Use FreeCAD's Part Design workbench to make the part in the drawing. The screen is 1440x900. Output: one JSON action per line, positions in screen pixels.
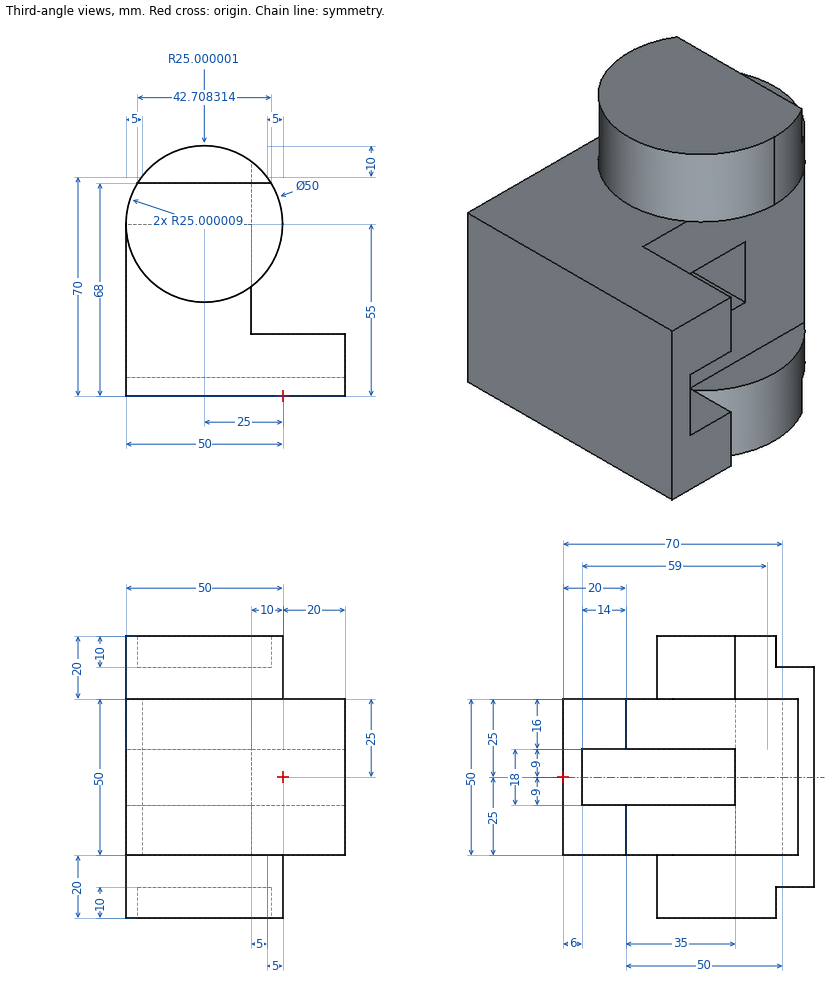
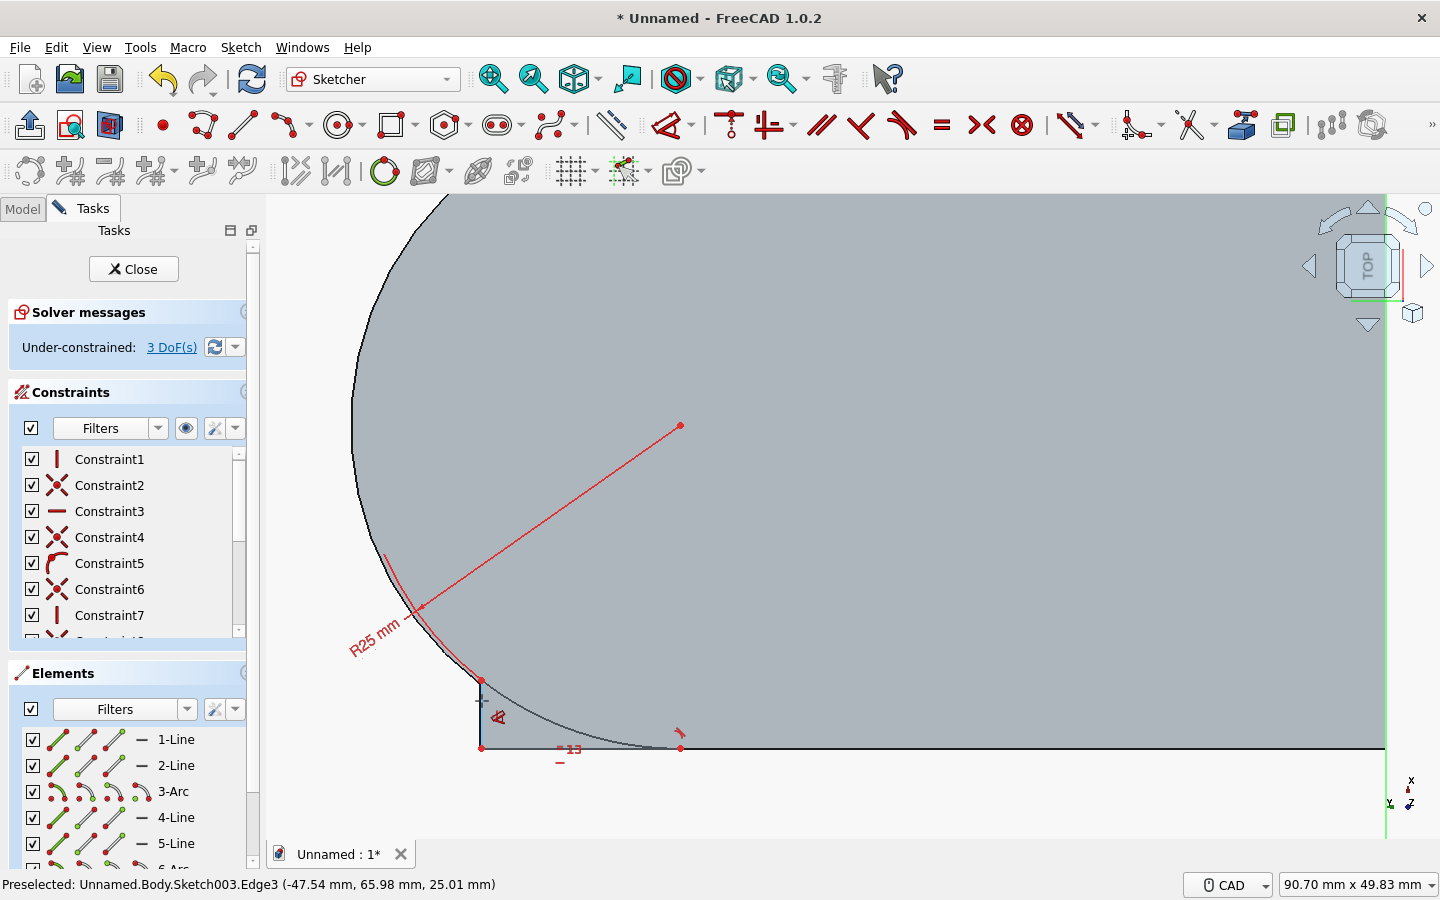
{"action": "left_click", "coordinate": [482, 701]}
{"action": "left_click", "coordinate": [448, 715]}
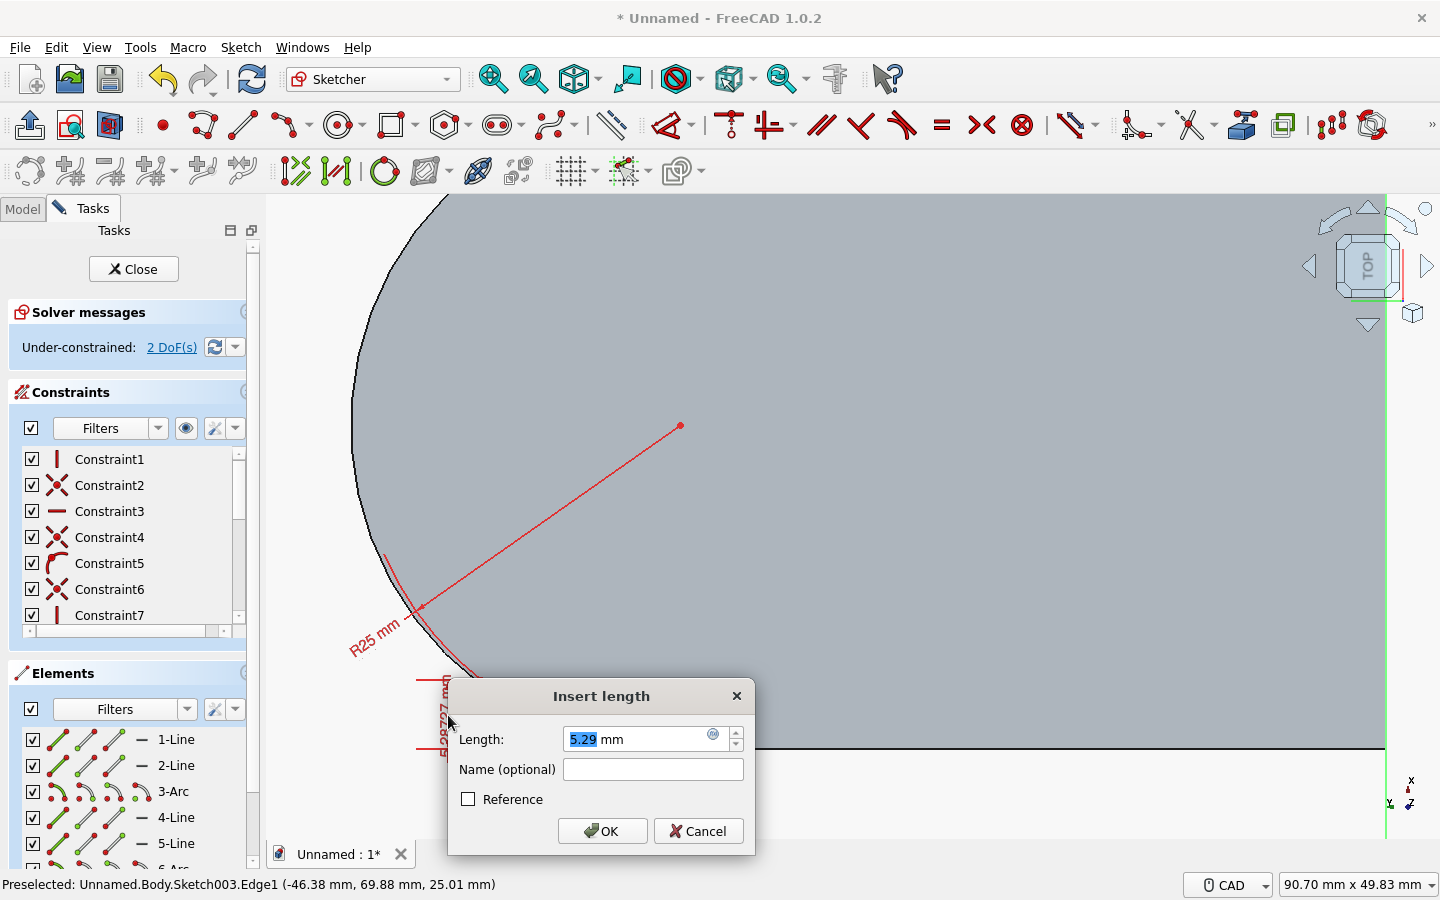
{"action": "type", "text": "5"}
{"action": "key", "text": "Return"}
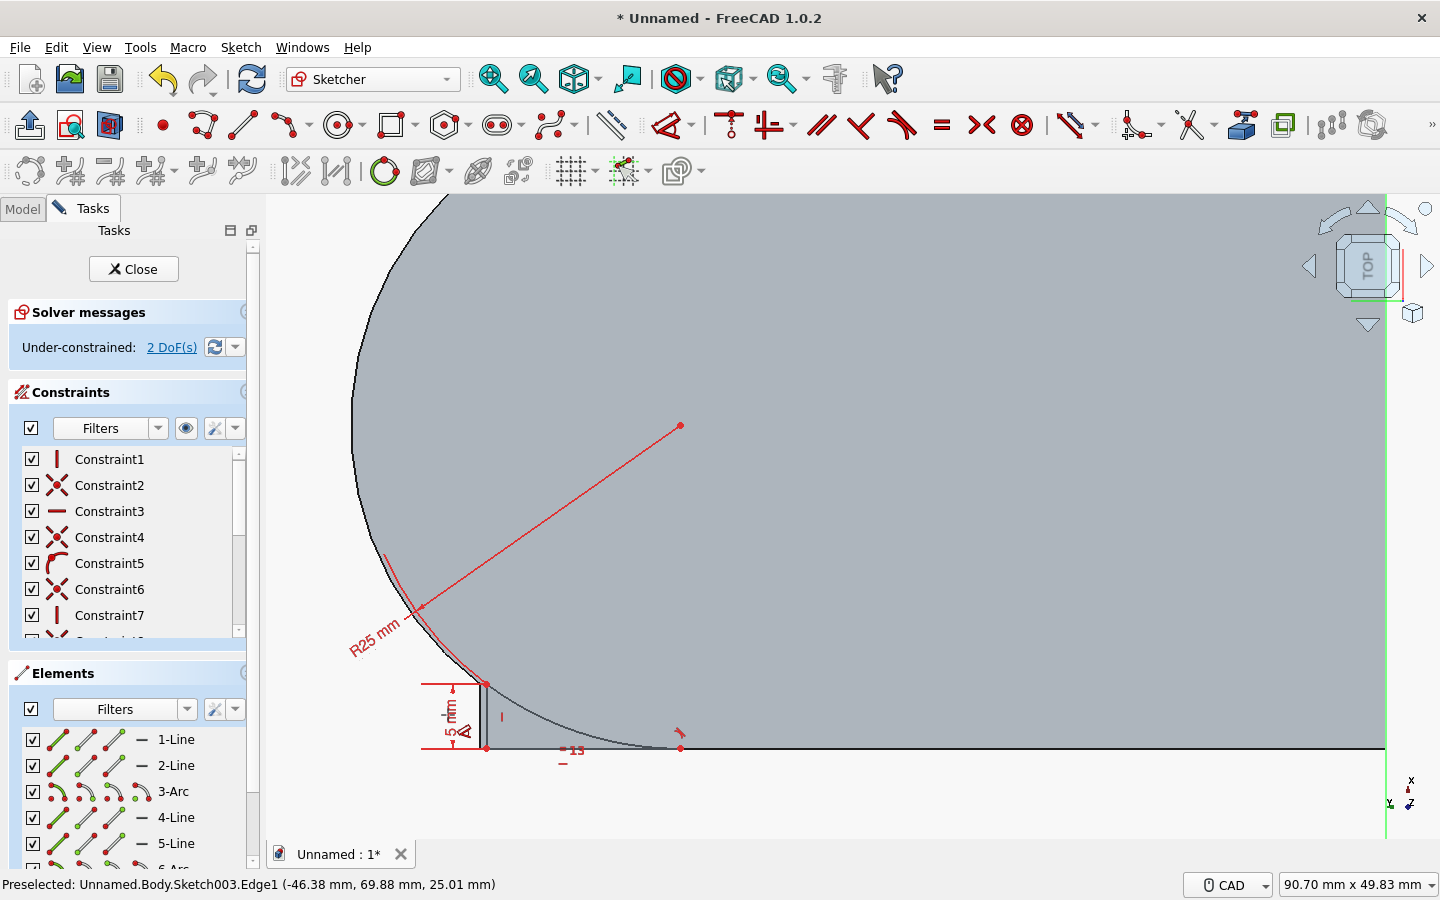
{"action": "scroll", "coordinate": [482, 702], "scroll_direction": "down", "scroll_amount": 2}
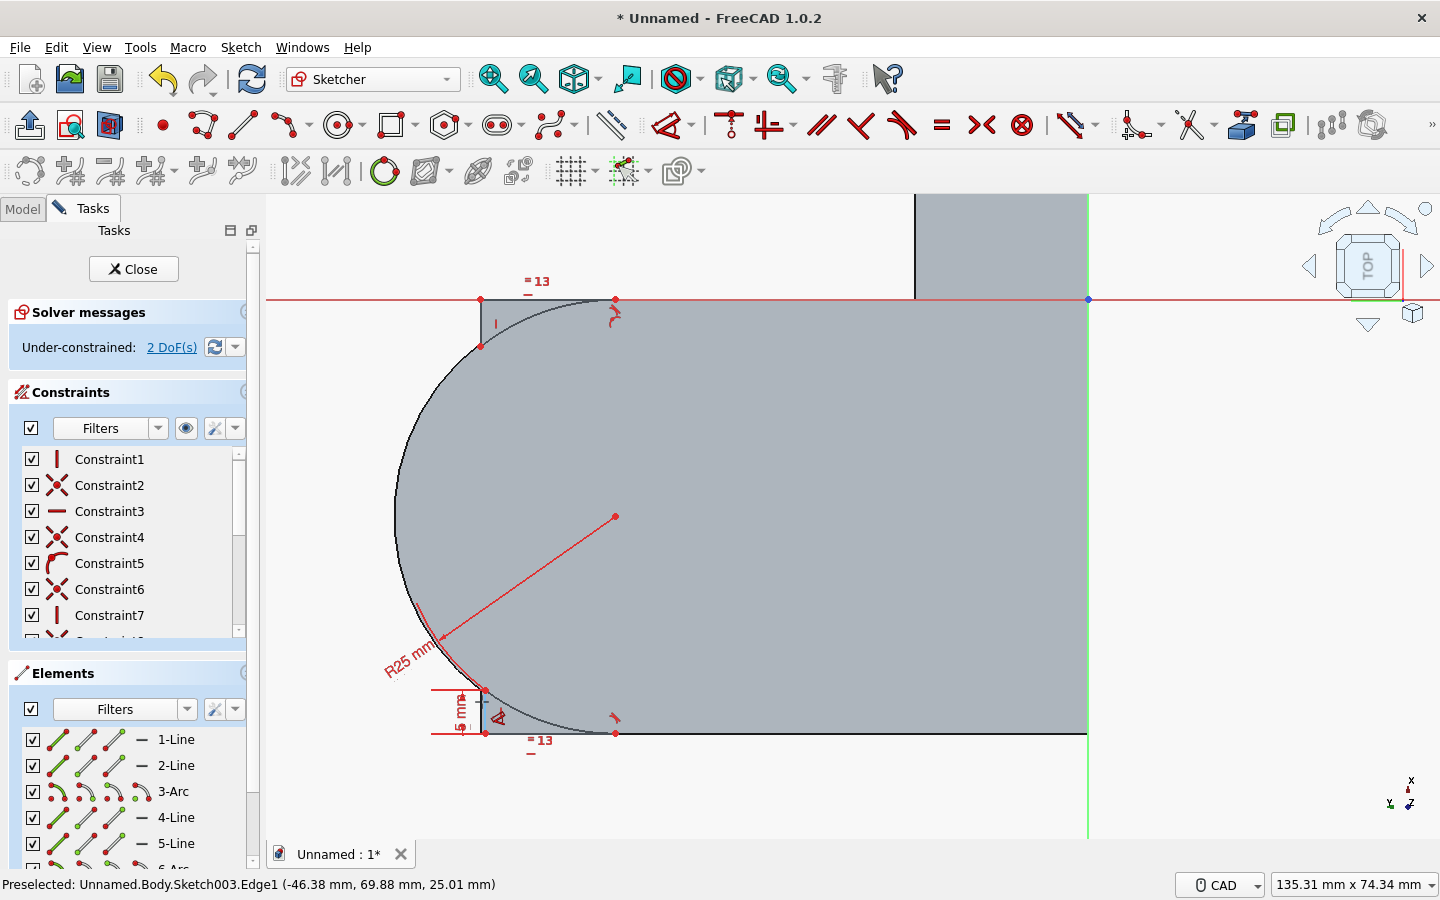
{"action": "left_click", "coordinate": [481, 314]}
{"action": "left_click", "coordinate": [447, 323]}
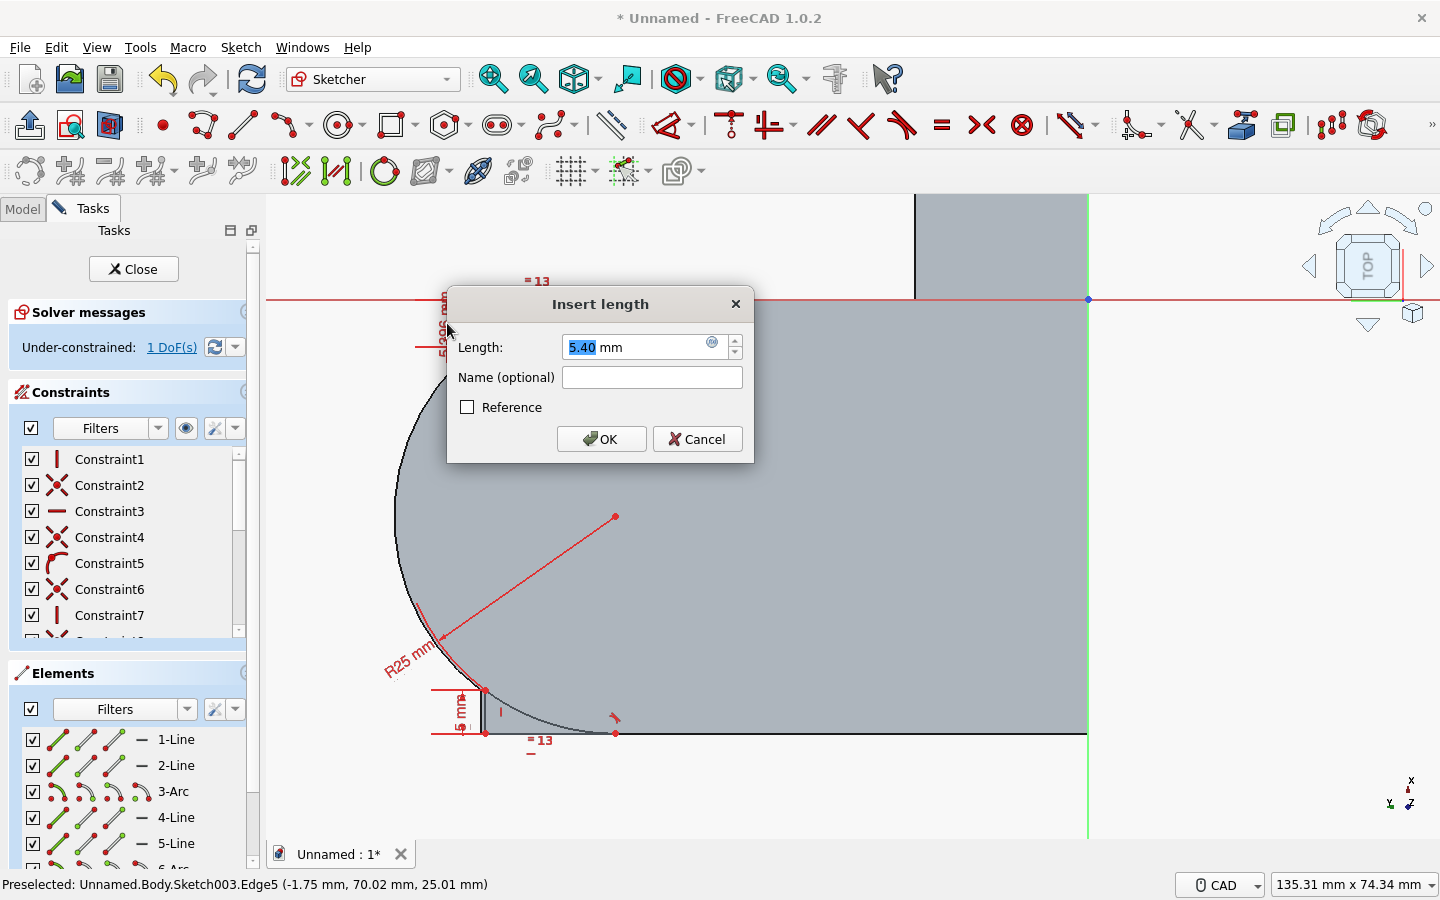
{"action": "type", "text": "5"}
{"action": "key", "text": "Return"}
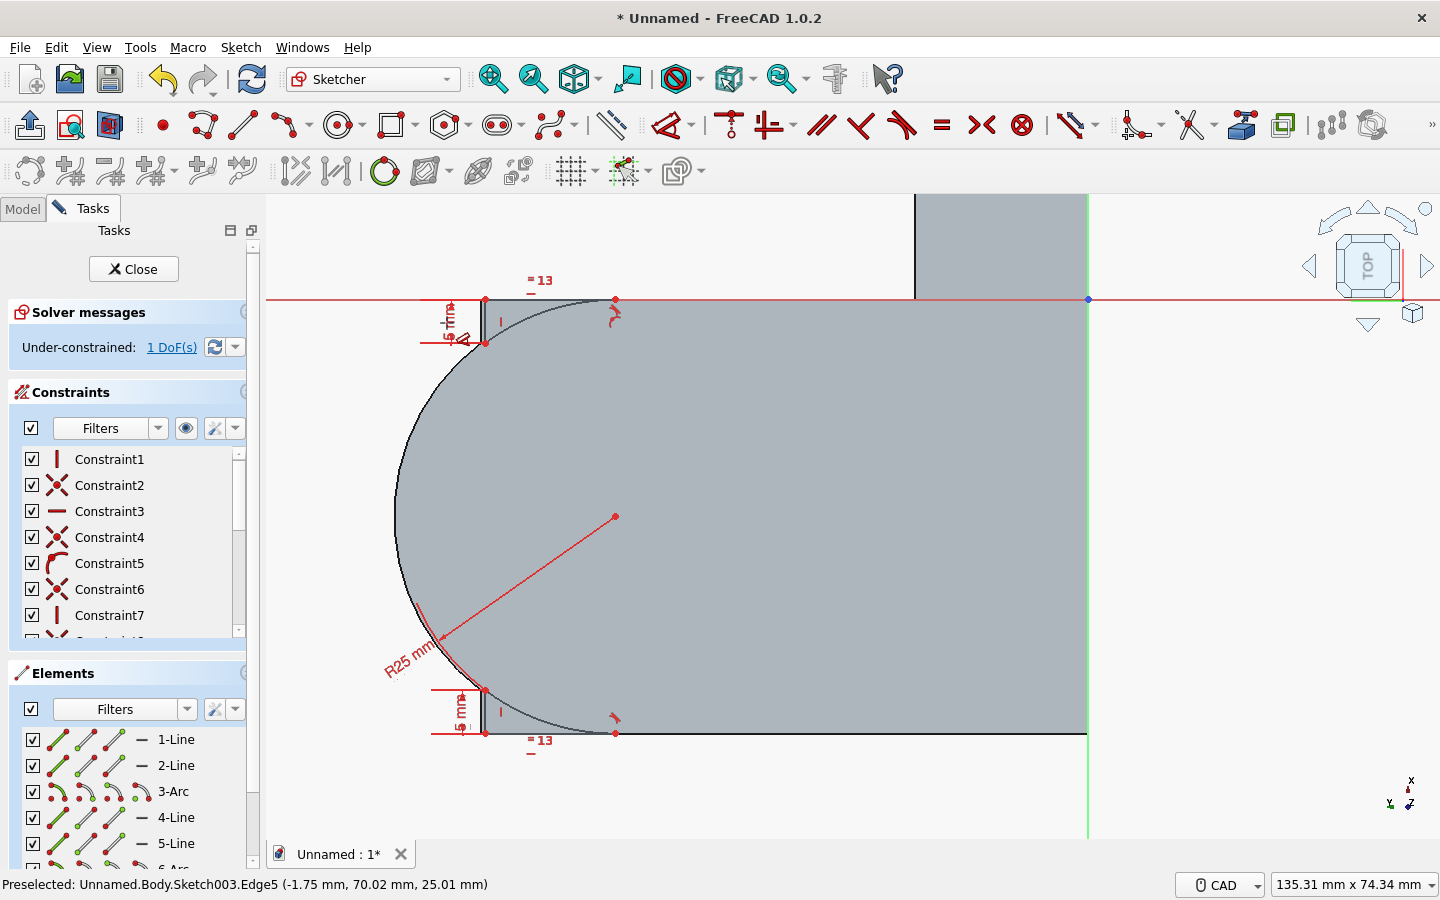
{"action": "left_click", "coordinate": [485, 690]}
{"action": "left_click", "coordinate": [787, 266]}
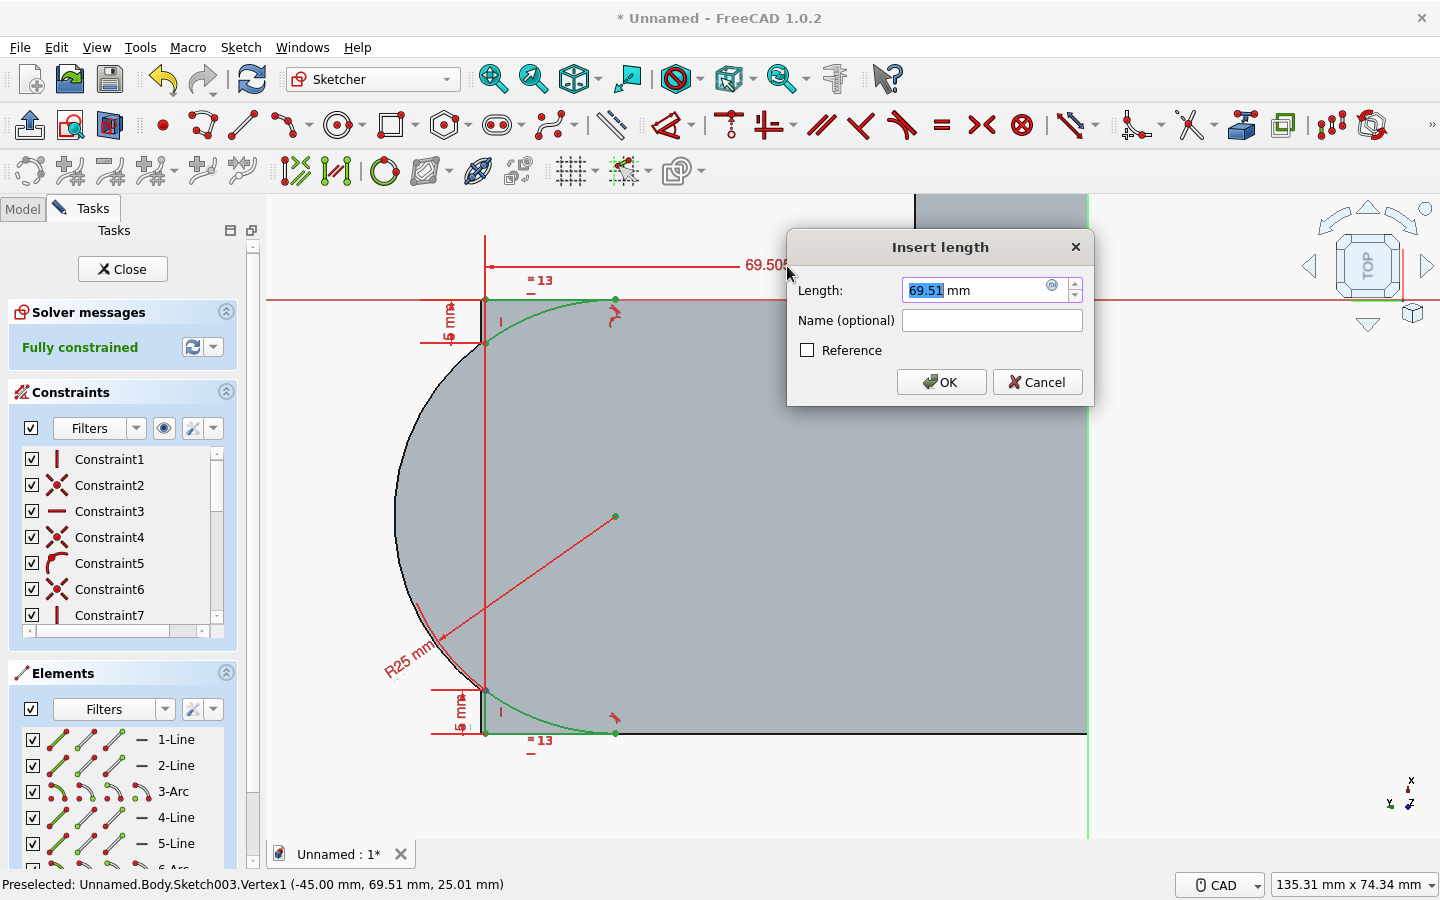
{"action": "type", "text": "70"}
{"action": "key", "text": "Return"}
{"action": "key", "text": "Escape"}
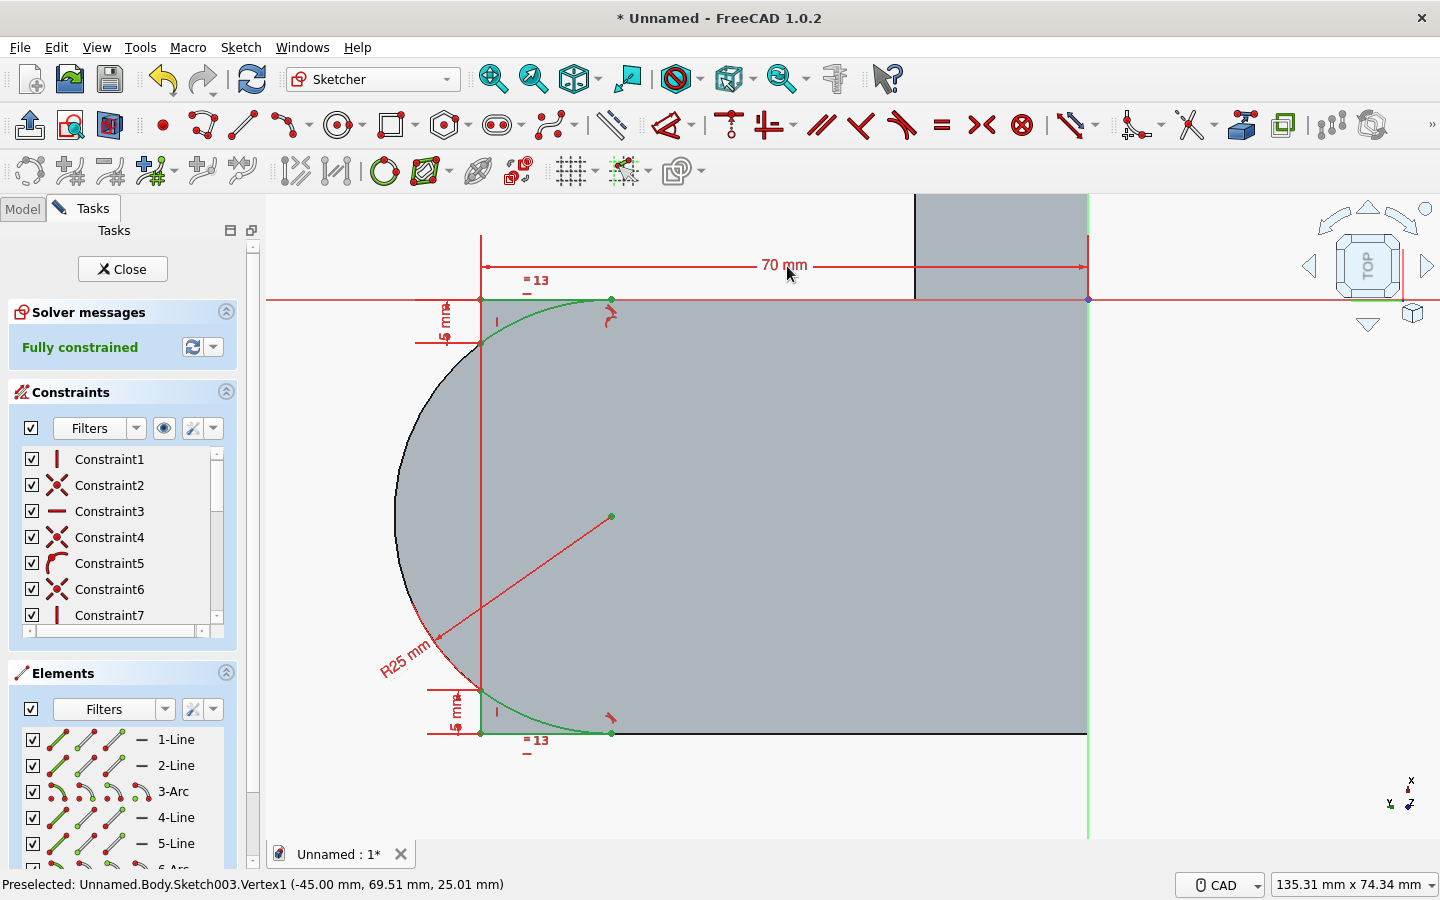
{"action": "left_click", "coordinate": [123, 269]}